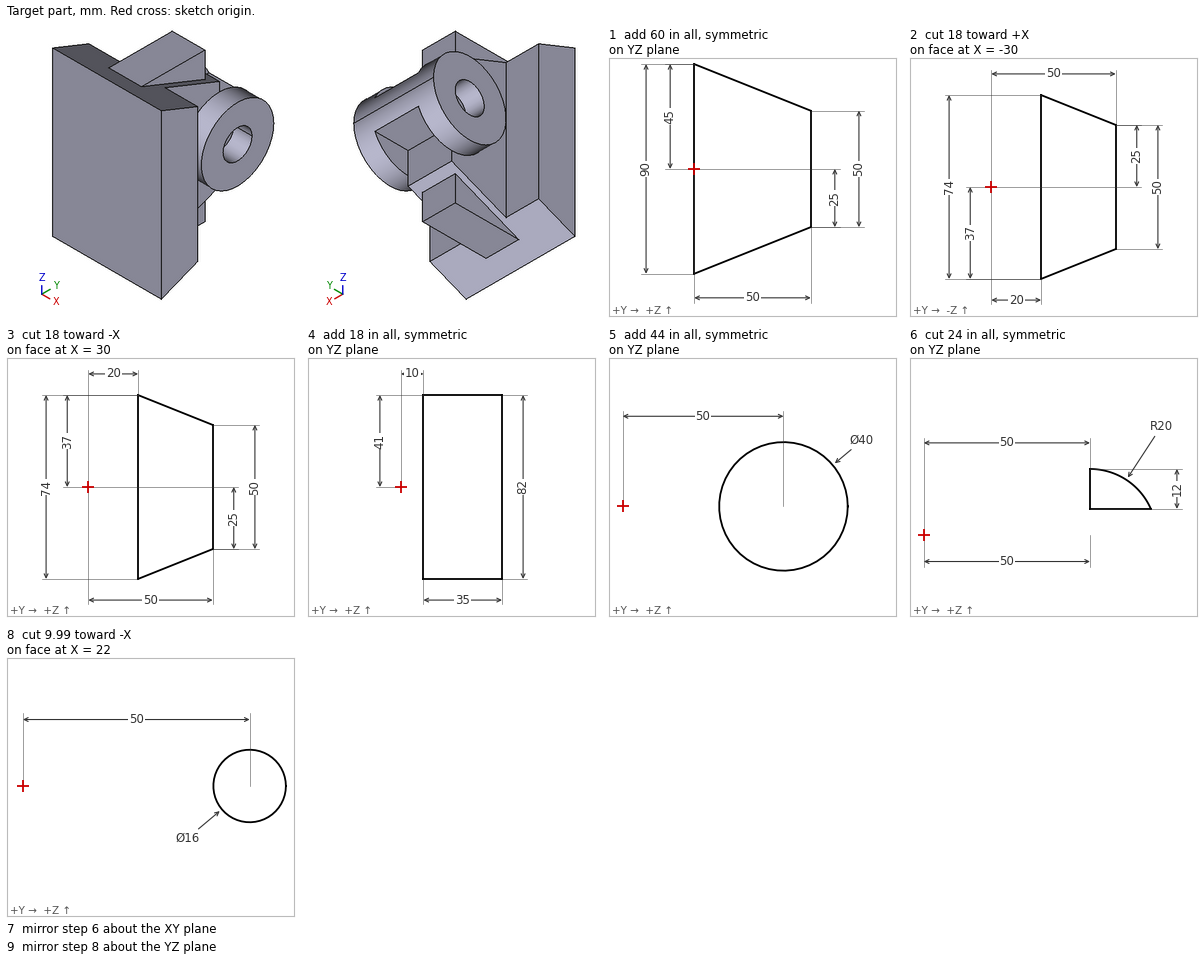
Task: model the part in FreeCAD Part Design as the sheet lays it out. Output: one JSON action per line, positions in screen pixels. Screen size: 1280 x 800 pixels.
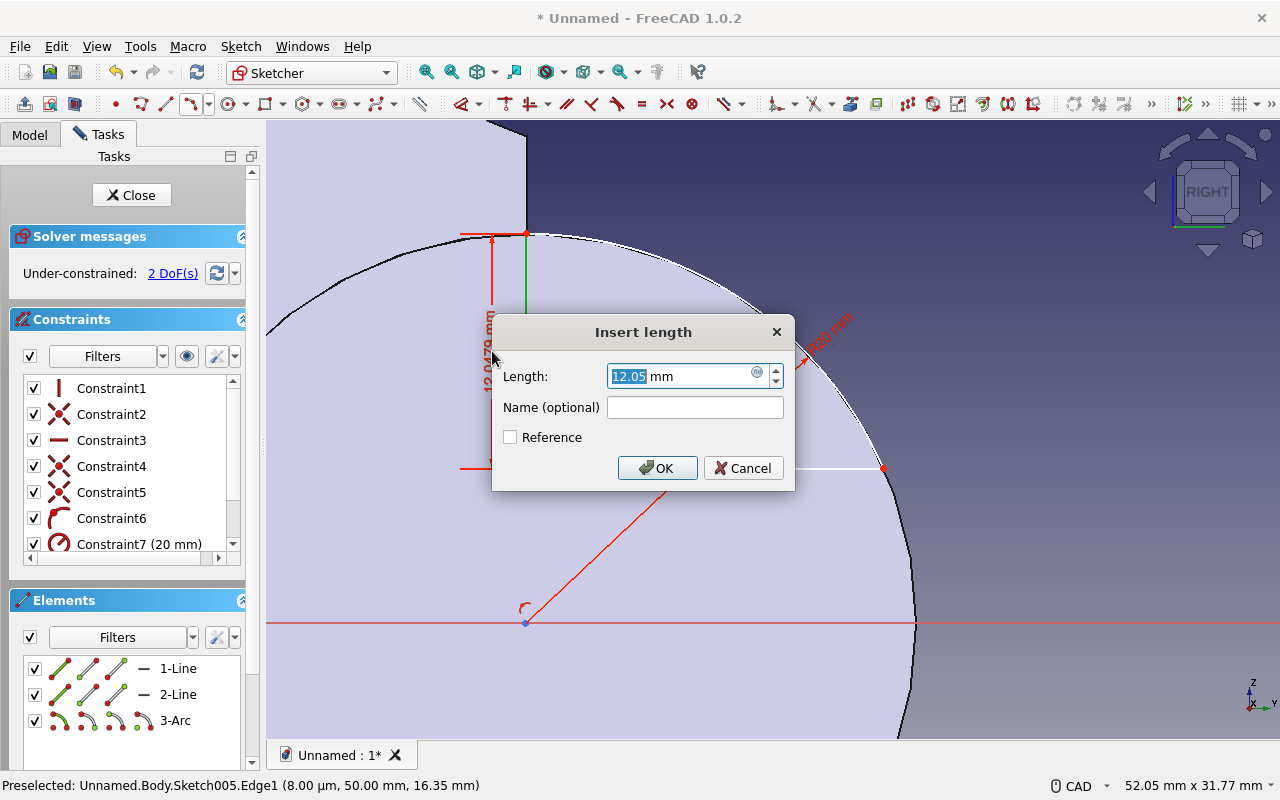
{"action": "type", "text": "12"}
{"action": "key", "text": "Return"}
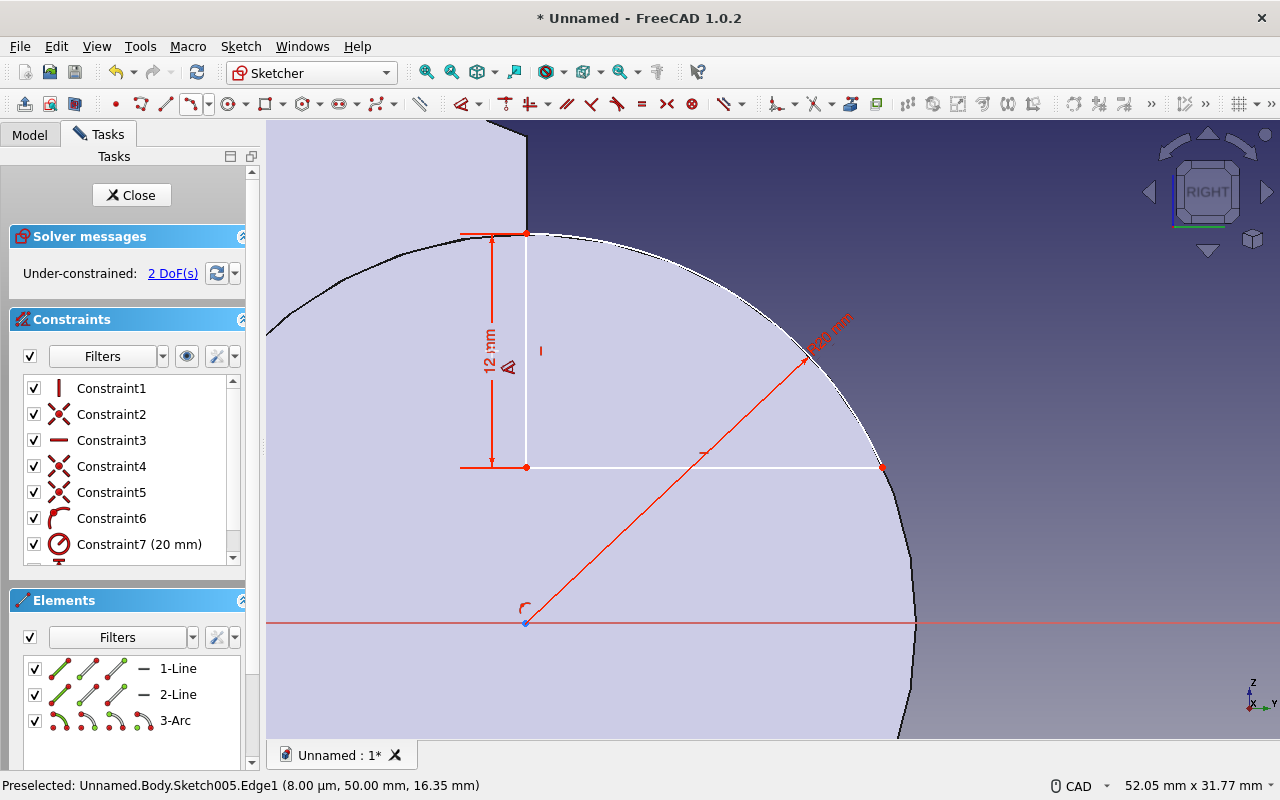
{"action": "left_click", "coordinate": [526, 234]}
{"action": "left_click", "coordinate": [410, 657]}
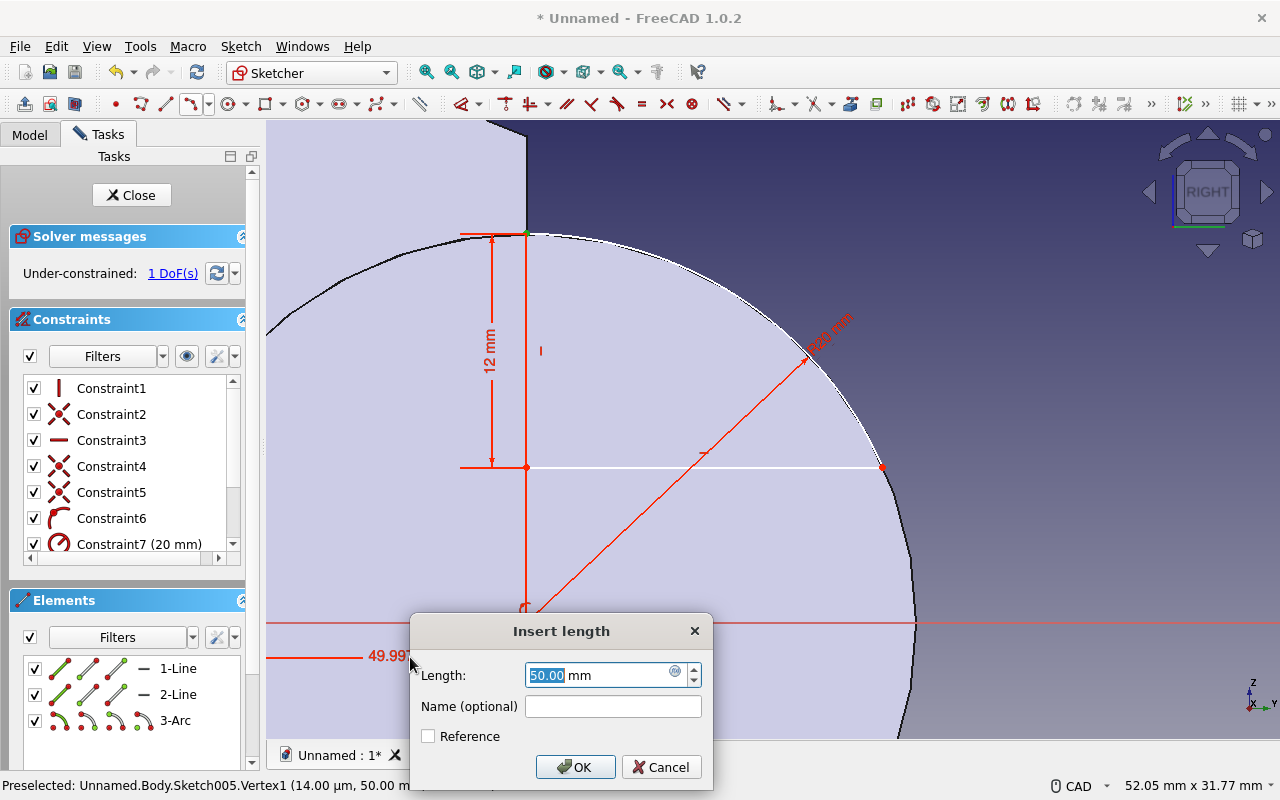
{"action": "type", "text": "50"}
{"action": "key", "text": "Return"}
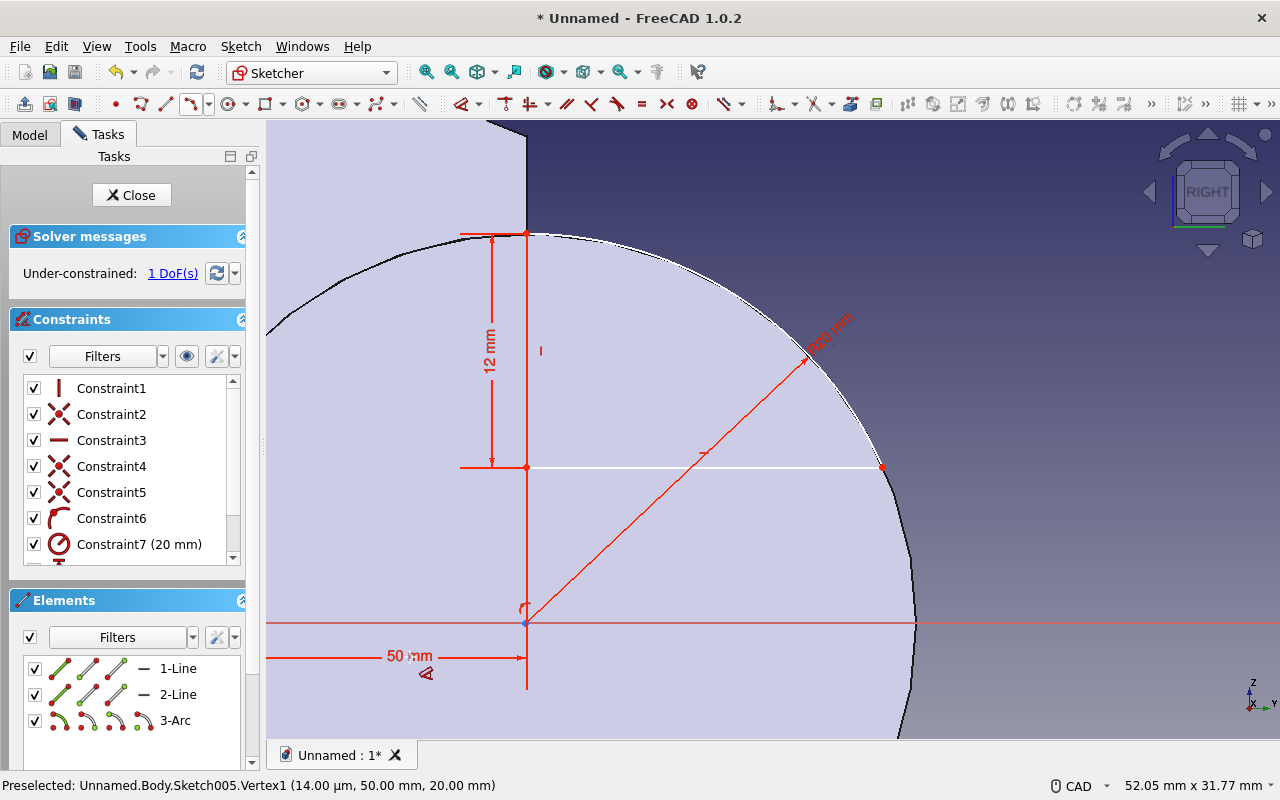
{"action": "left_click", "coordinate": [526, 623]}
{"action": "left_click", "coordinate": [329, 657]}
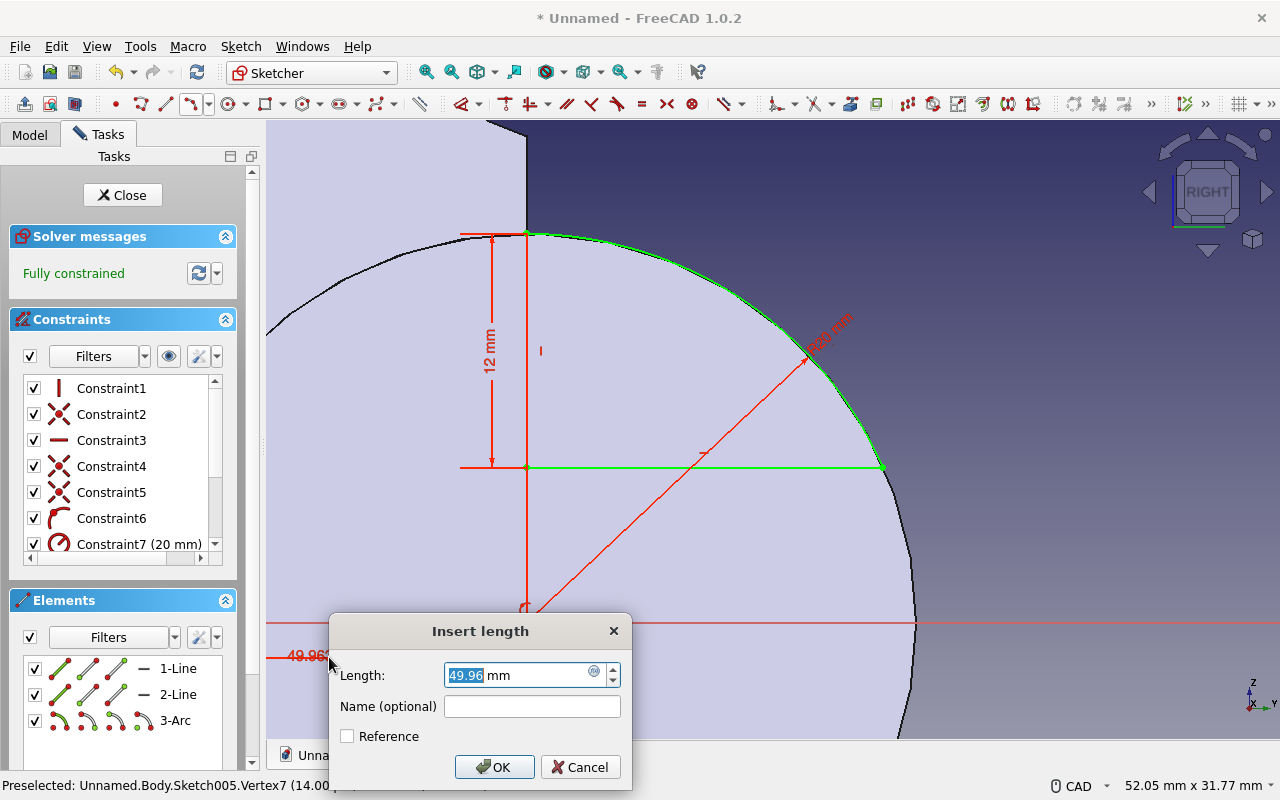
{"action": "type", "text": "50"}
{"action": "key", "text": "Return"}
{"action": "key", "text": "Escape"}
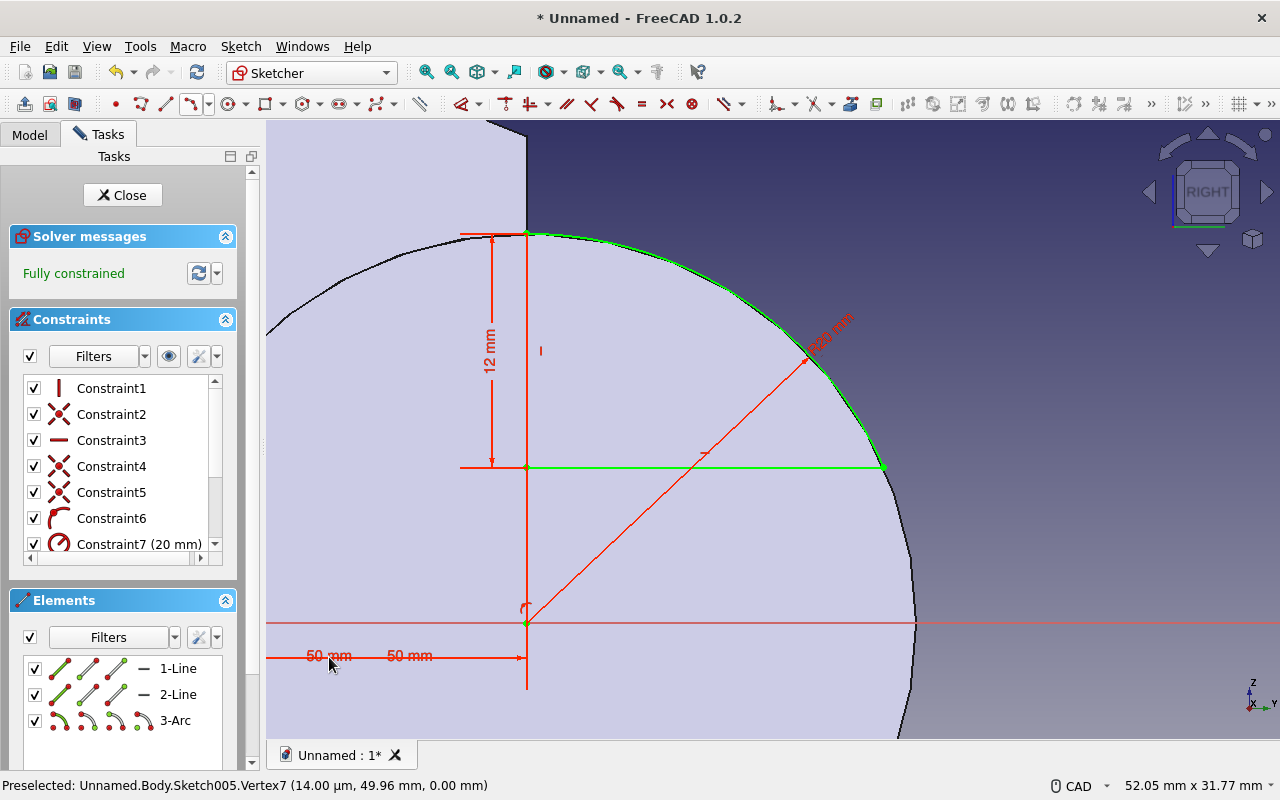
{"action": "left_click", "coordinate": [123, 195]}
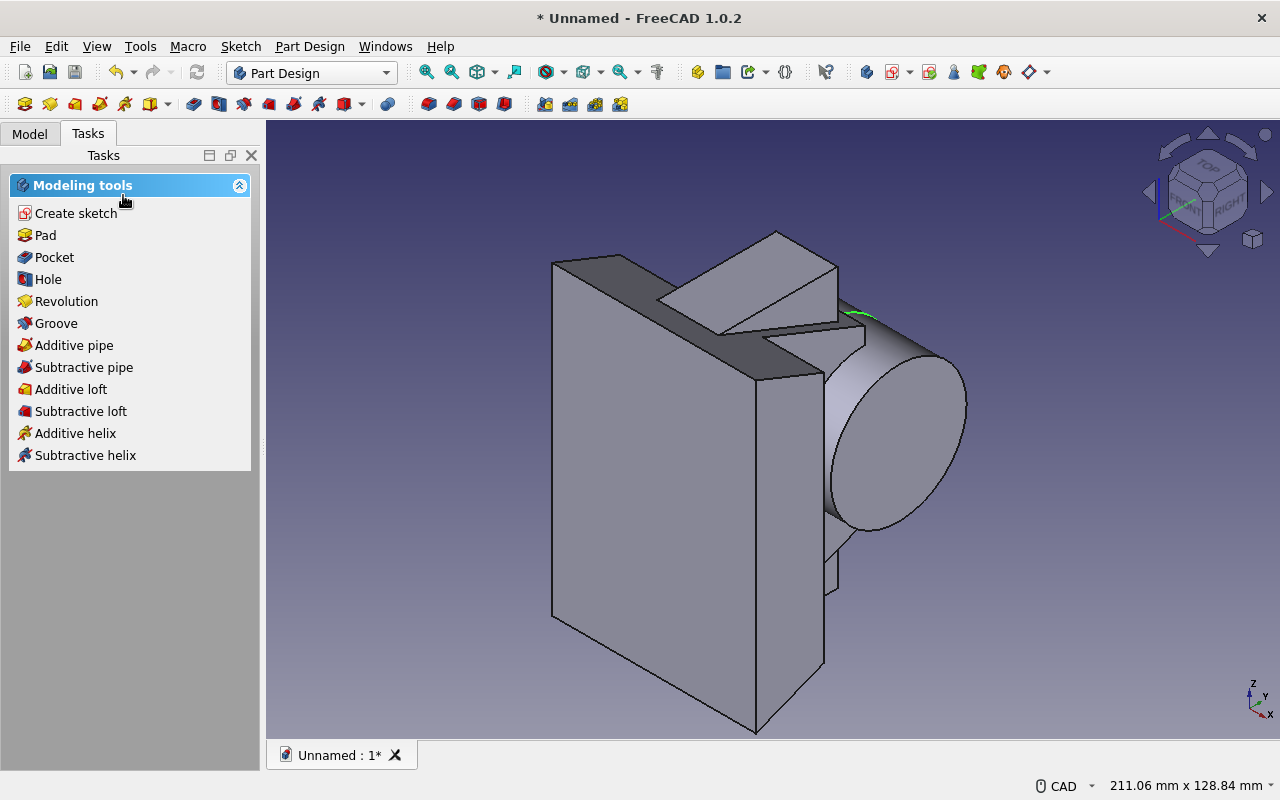
{"action": "left_click", "coordinate": [194, 104]}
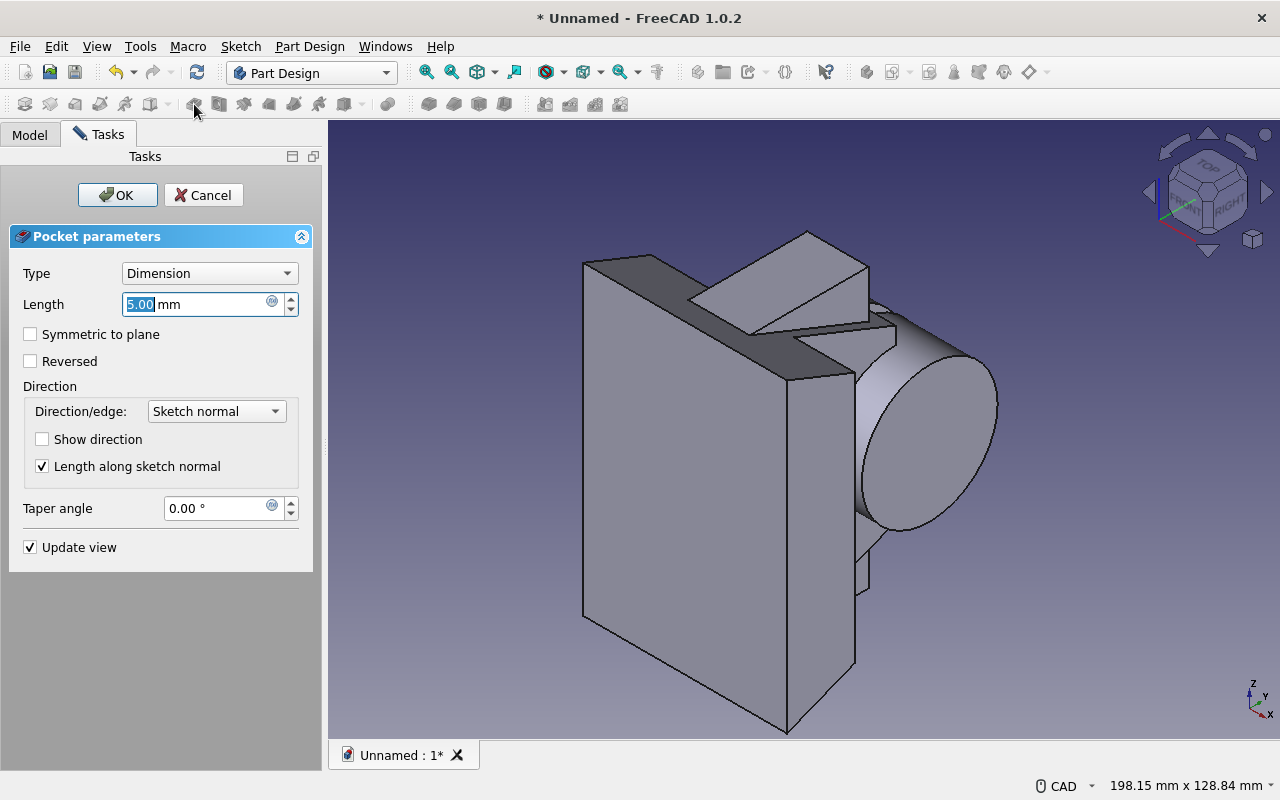
{"action": "type", "text": "24"}
{"action": "key", "text": "Tab"}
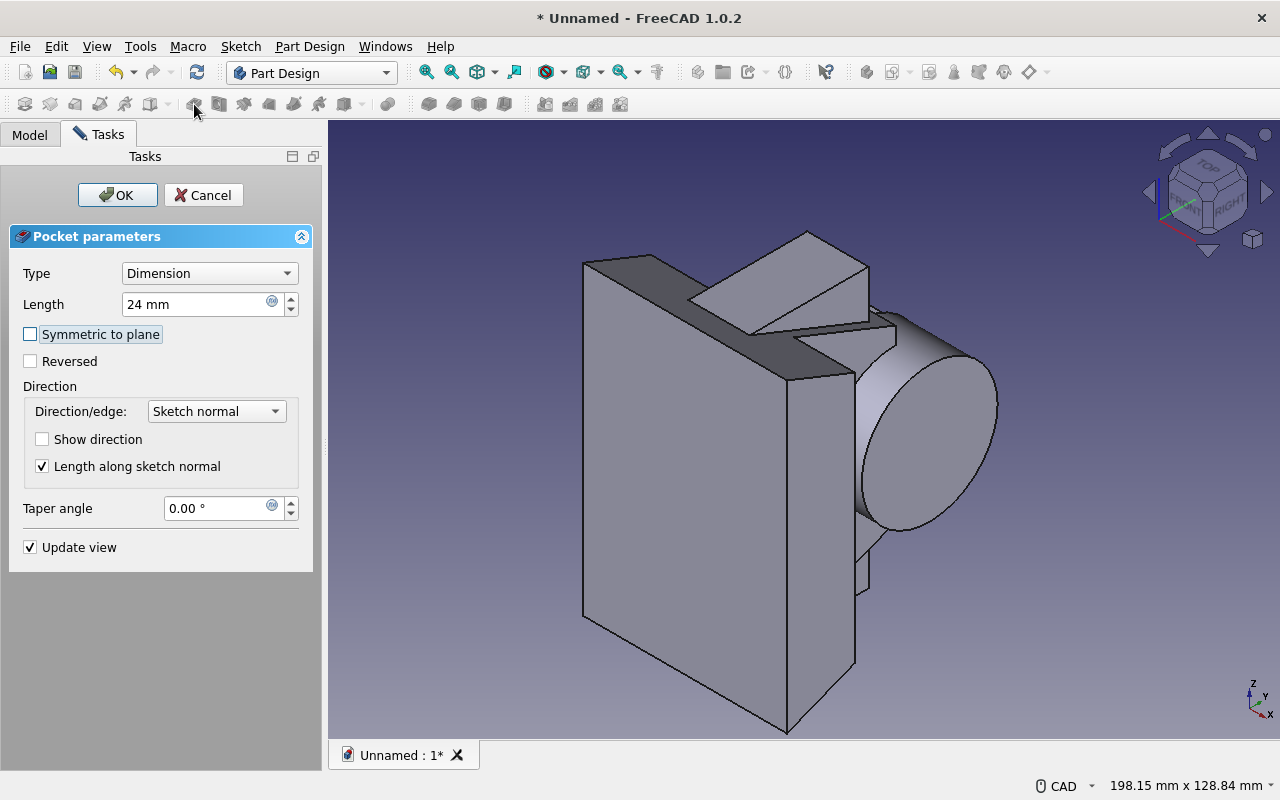
{"action": "left_click", "coordinate": [31, 334]}